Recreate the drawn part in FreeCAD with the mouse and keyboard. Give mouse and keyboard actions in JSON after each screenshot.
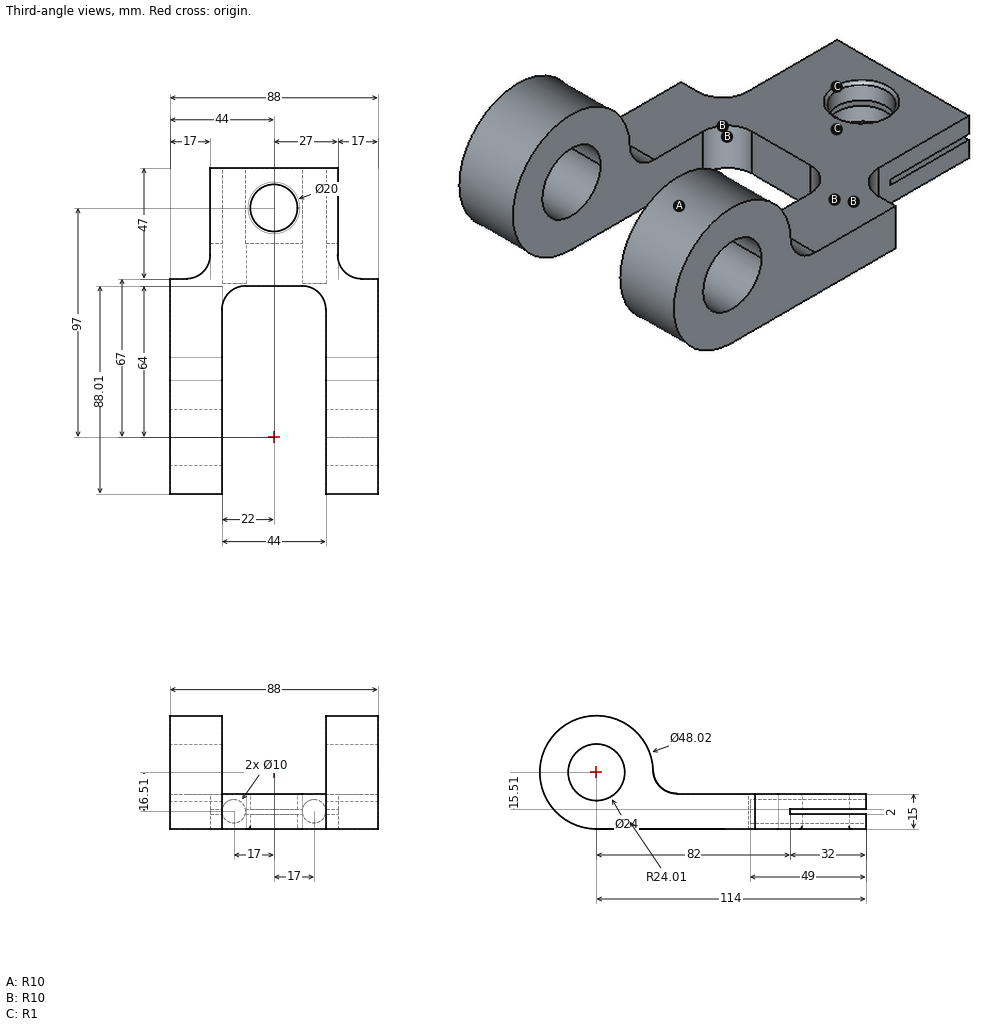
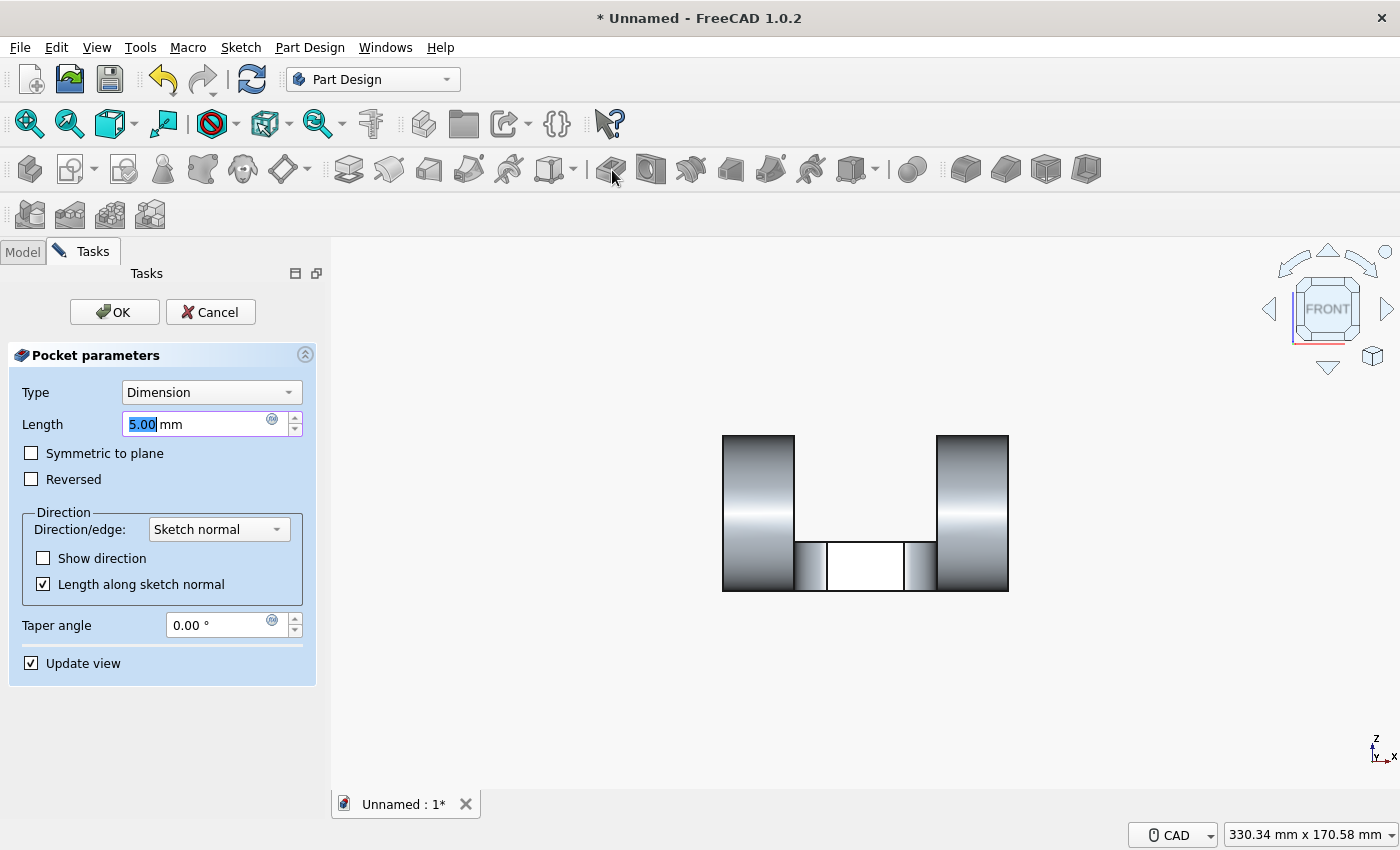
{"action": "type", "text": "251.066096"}
{"action": "key", "text": "Tab"}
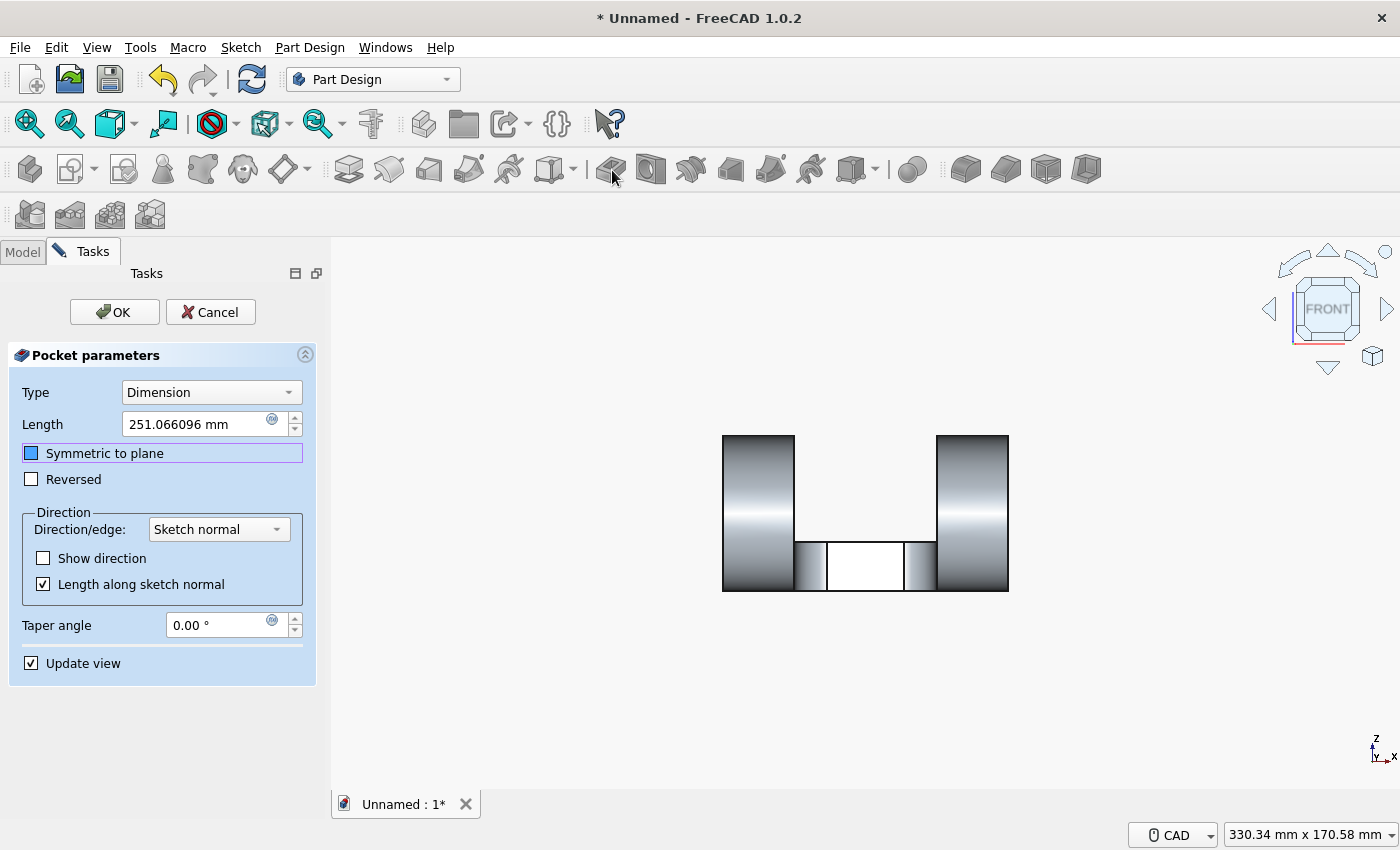
{"action": "left_click", "coordinate": [30, 453]}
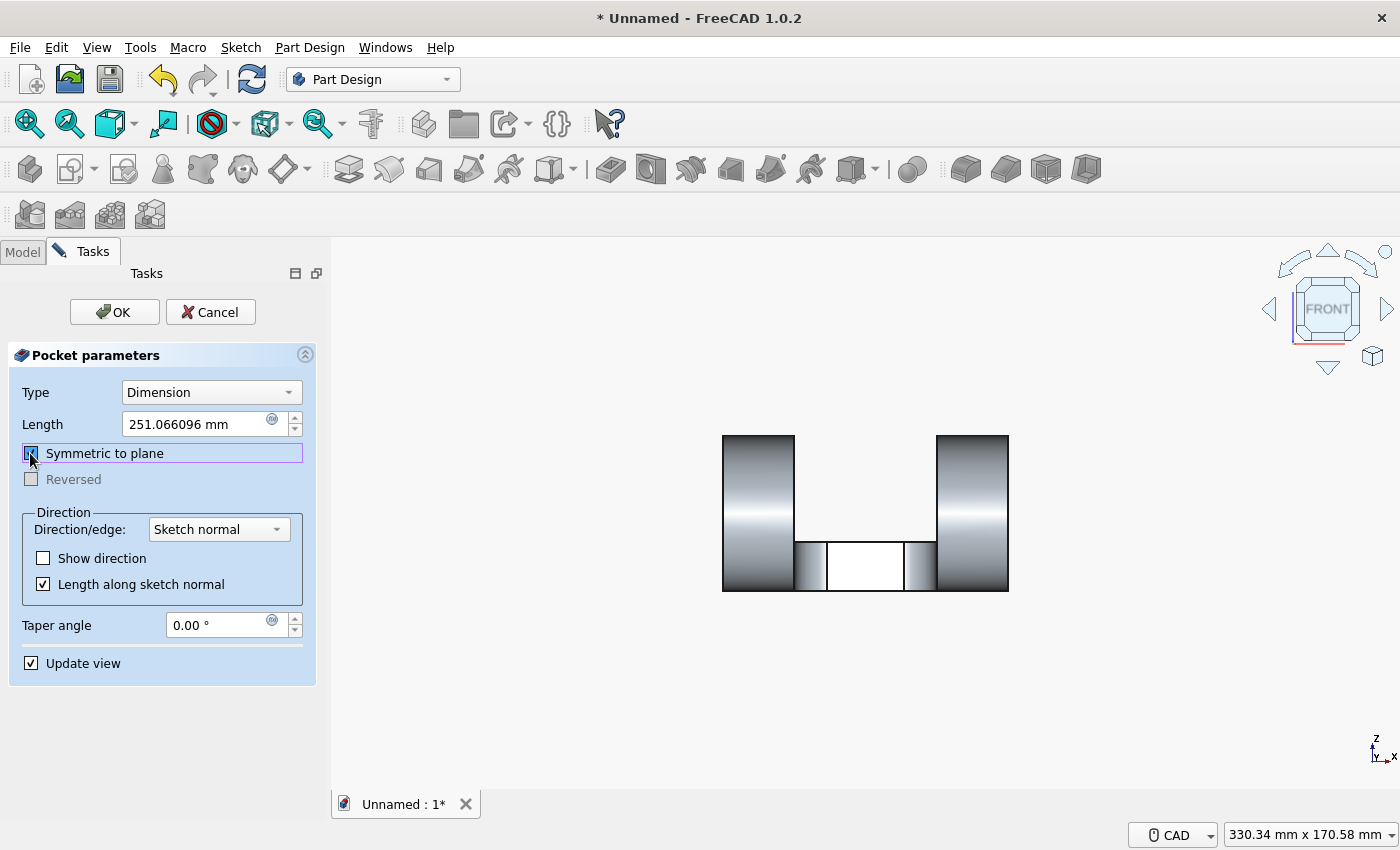
{"action": "left_click", "coordinate": [115, 312]}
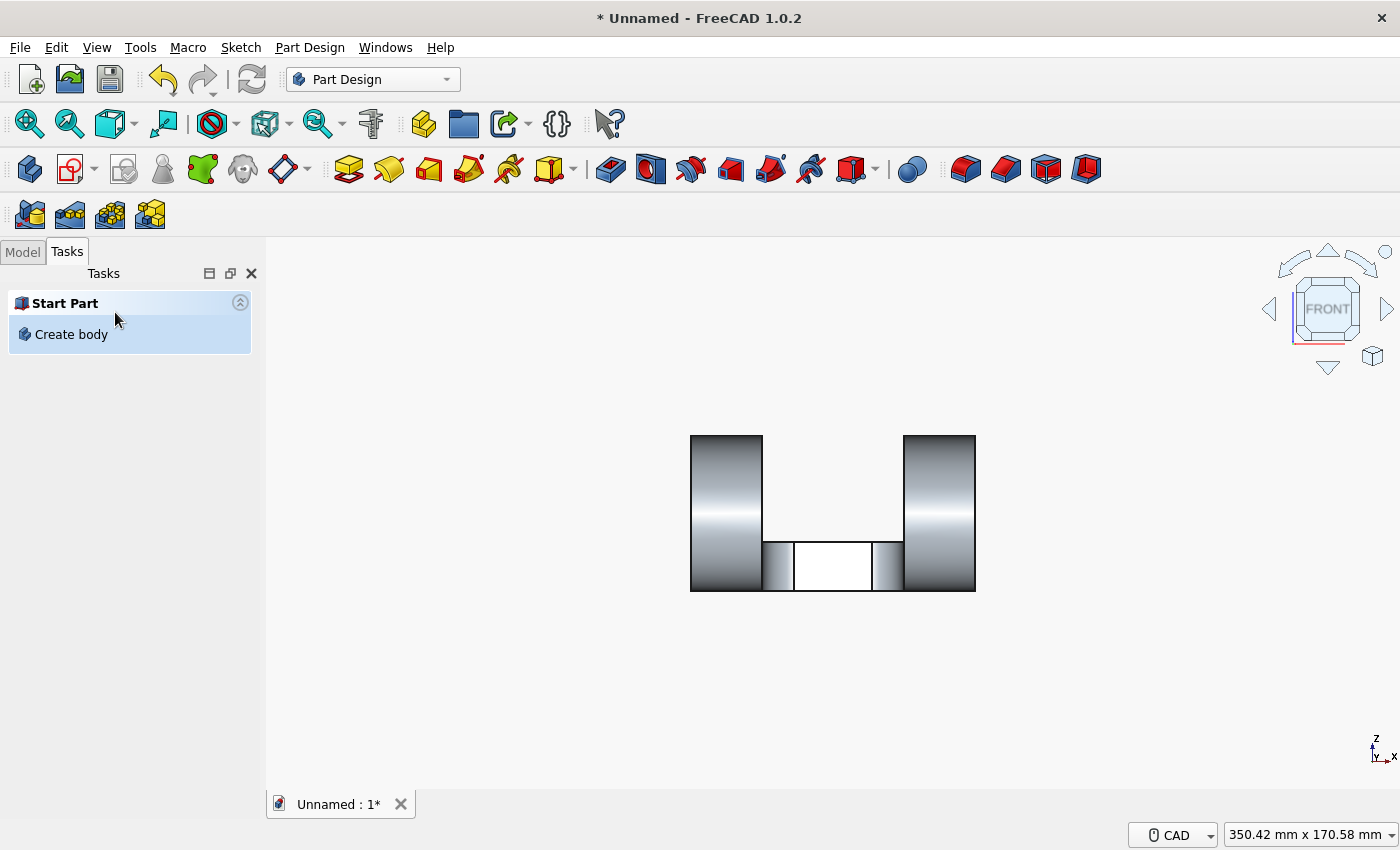
{"action": "left_click", "coordinate": [30, 124]}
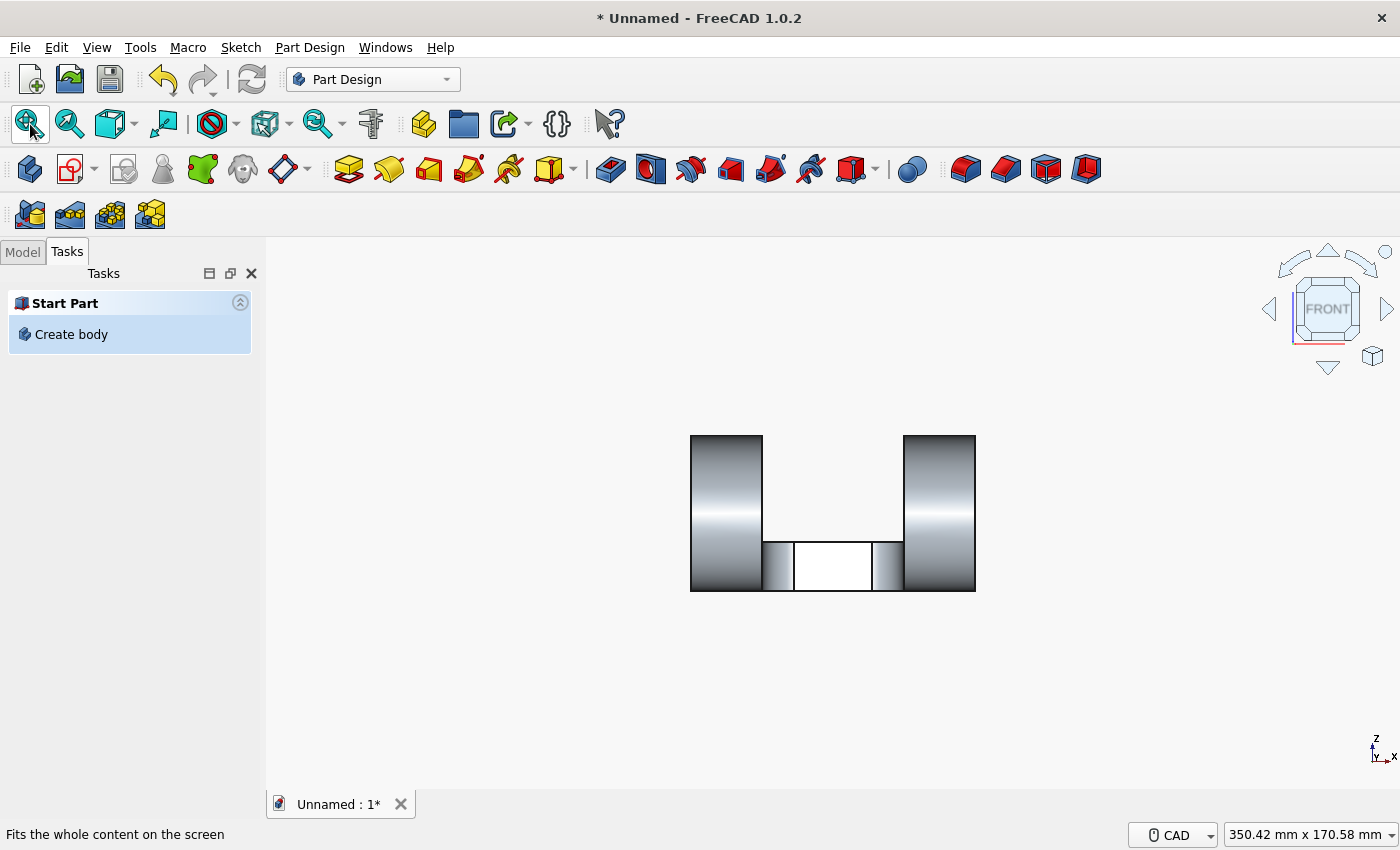
{"action": "key", "text": "0"}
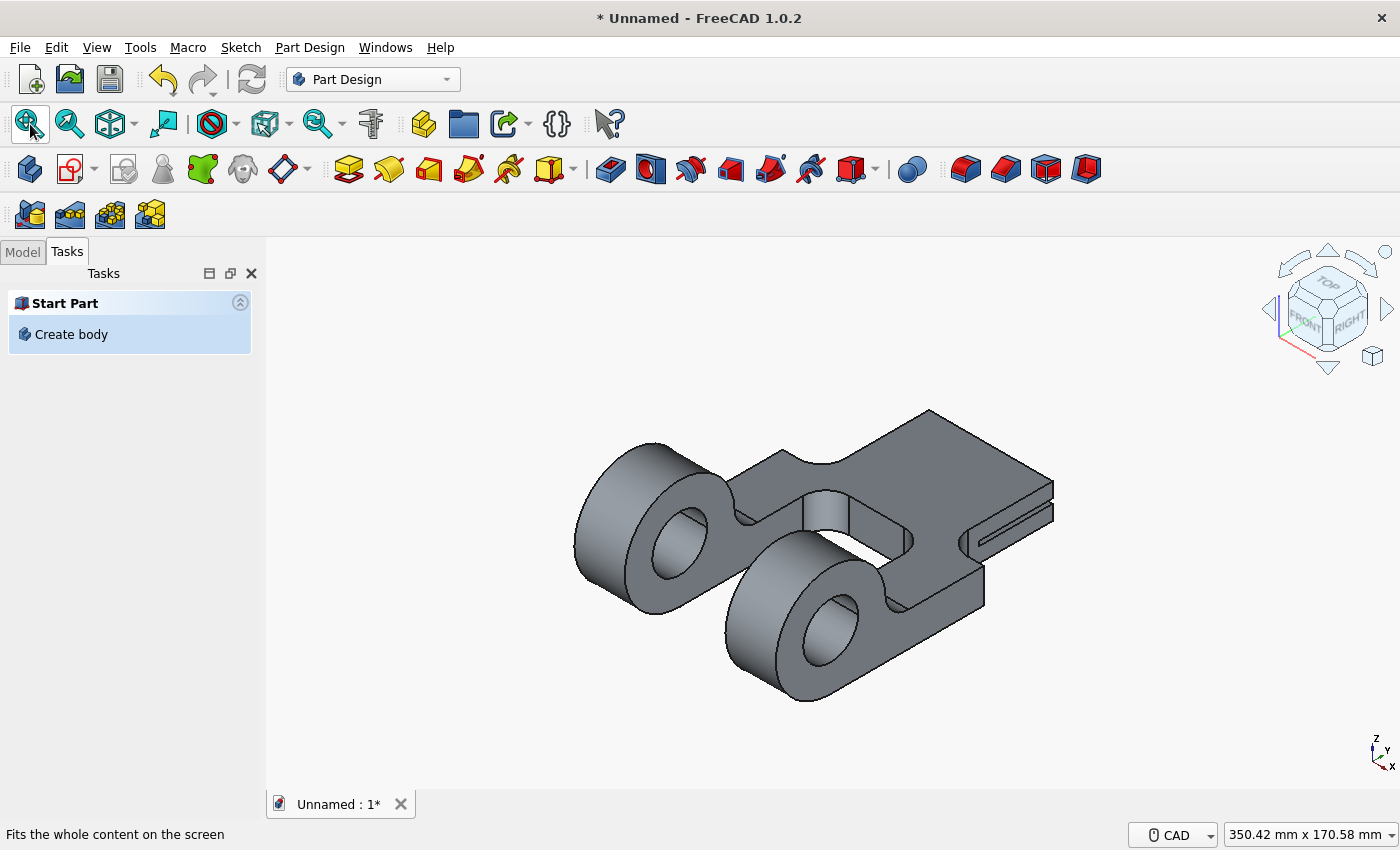
{"action": "left_click", "coordinate": [926, 482]}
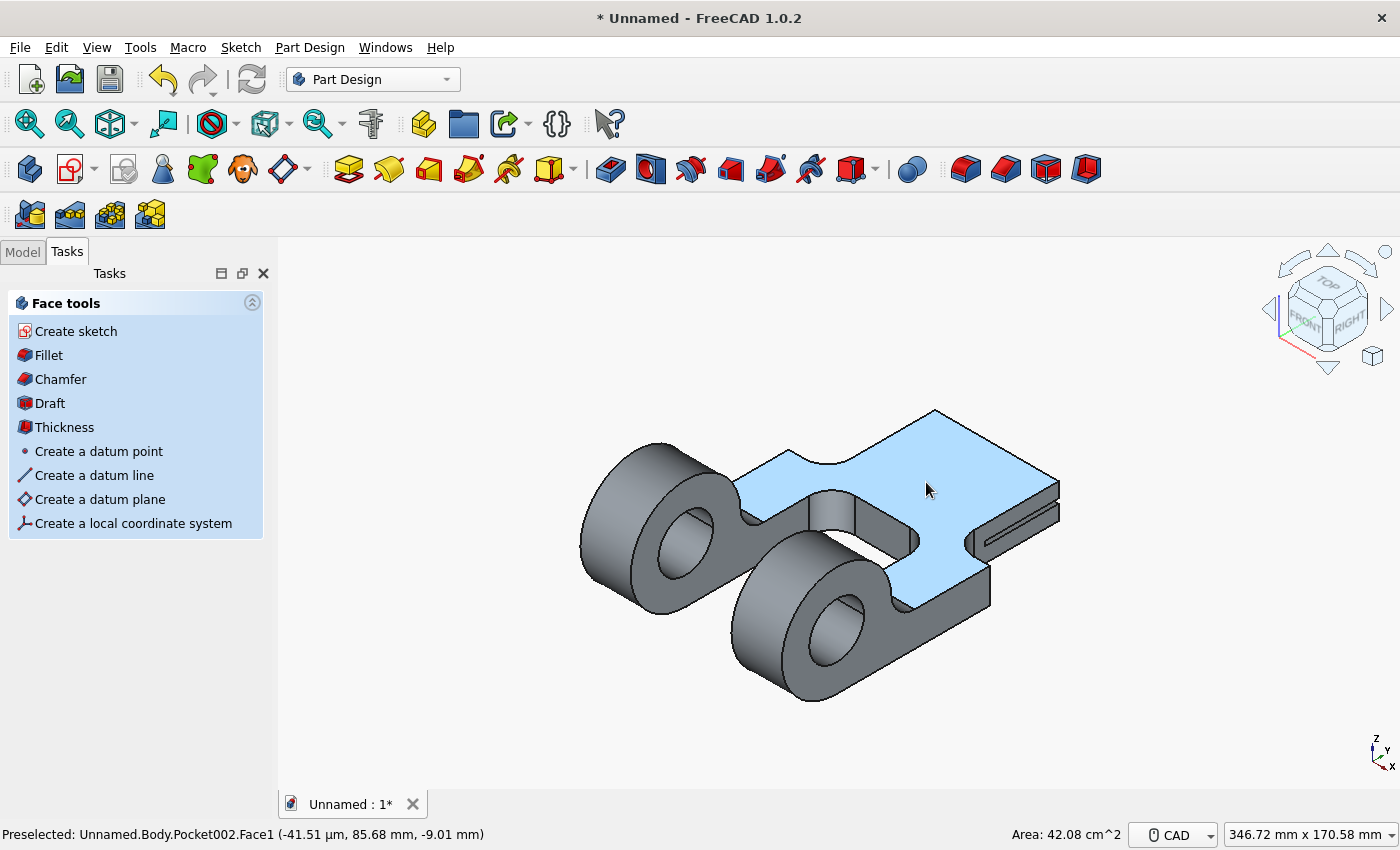
{"action": "left_click", "coordinate": [70, 170]}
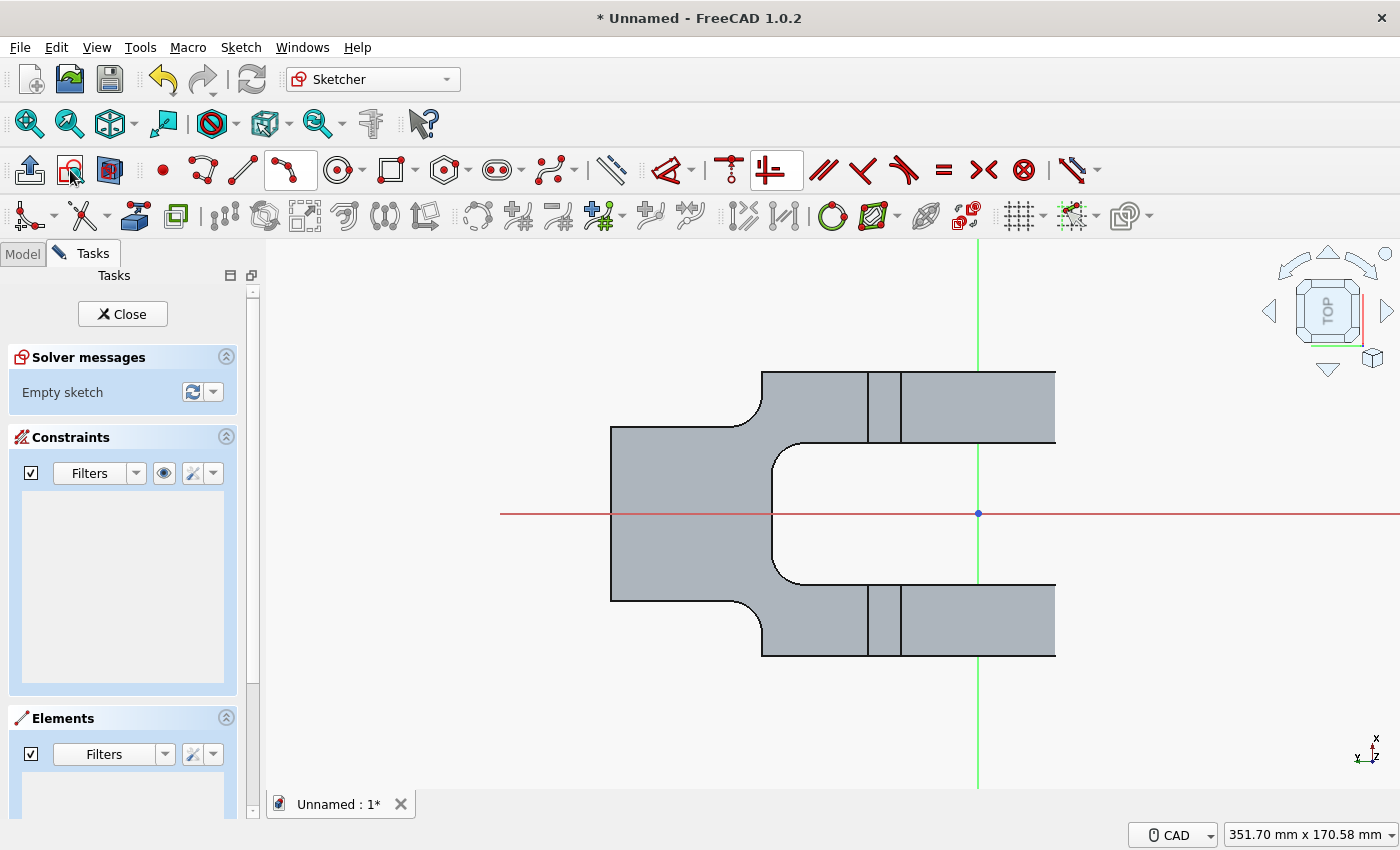
{"action": "left_click", "coordinate": [110, 170]}